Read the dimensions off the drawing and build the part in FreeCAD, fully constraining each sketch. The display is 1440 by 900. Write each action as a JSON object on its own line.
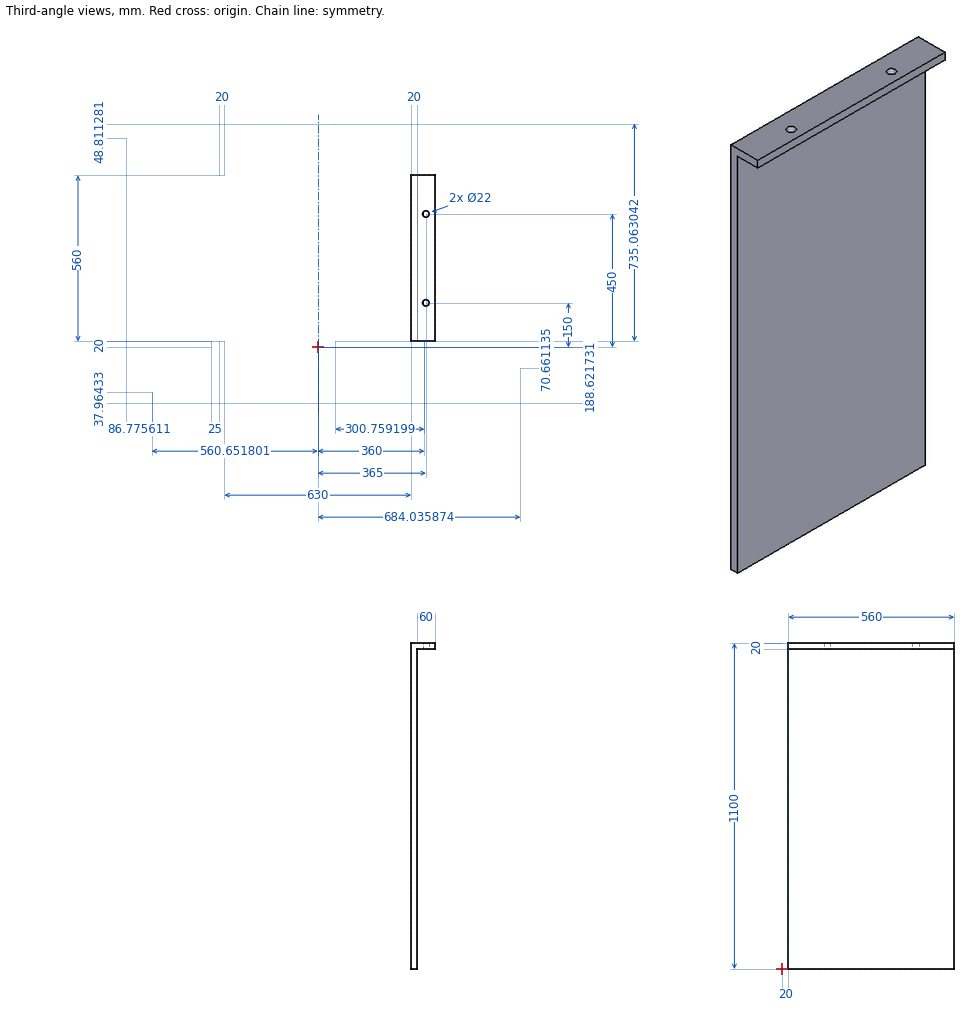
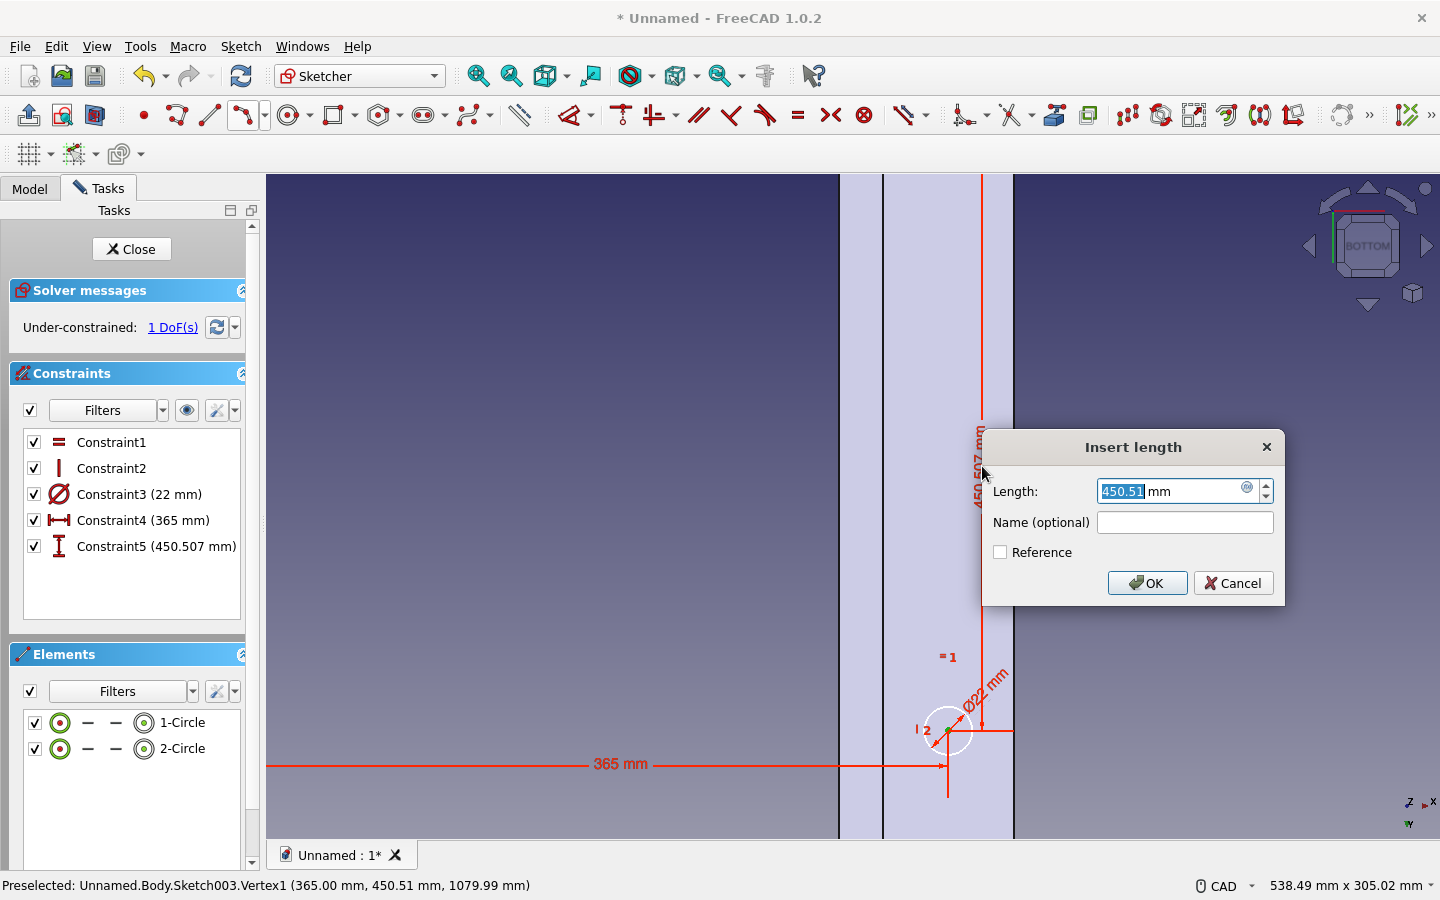
{"action": "type", "text": "450"}
{"action": "key", "text": "Return"}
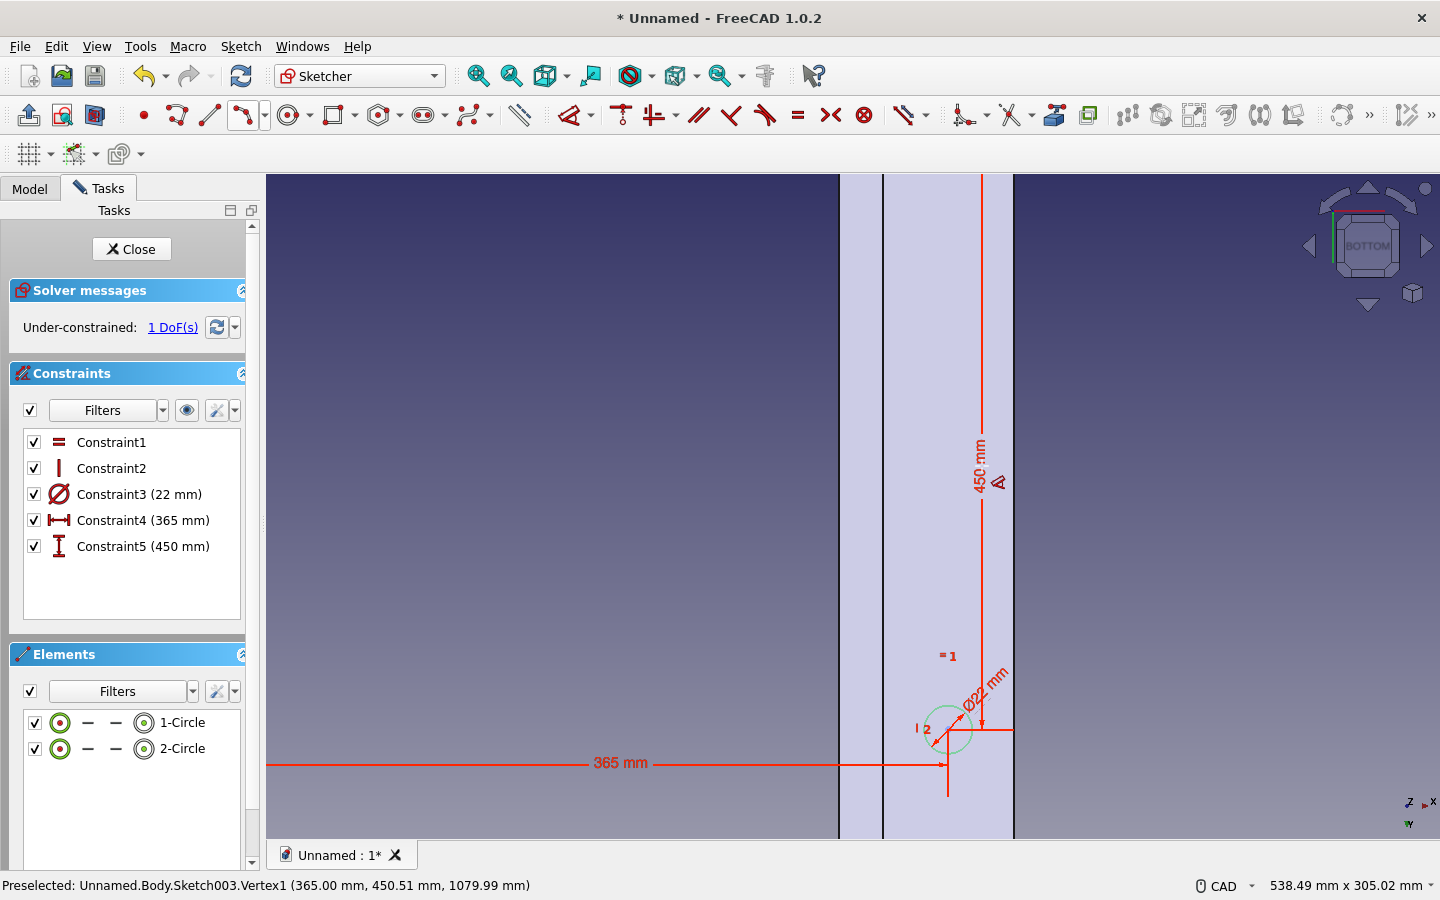
{"action": "scroll", "coordinate": [966, 715], "scroll_direction": "down", "scroll_amount": 4}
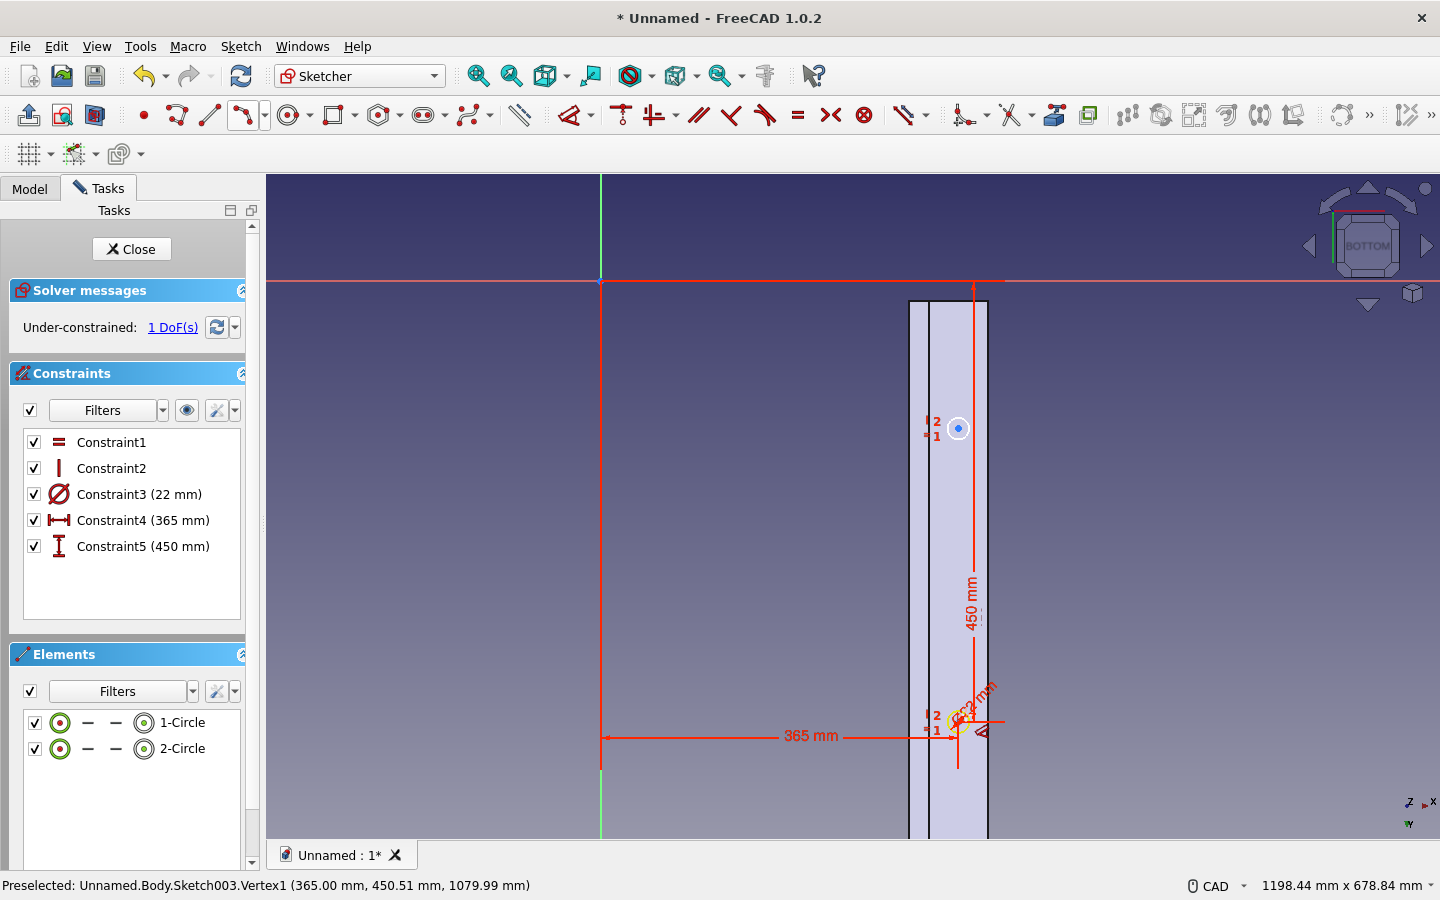
{"action": "left_click", "coordinate": [958, 429]}
{"action": "left_click", "coordinate": [567, 355]}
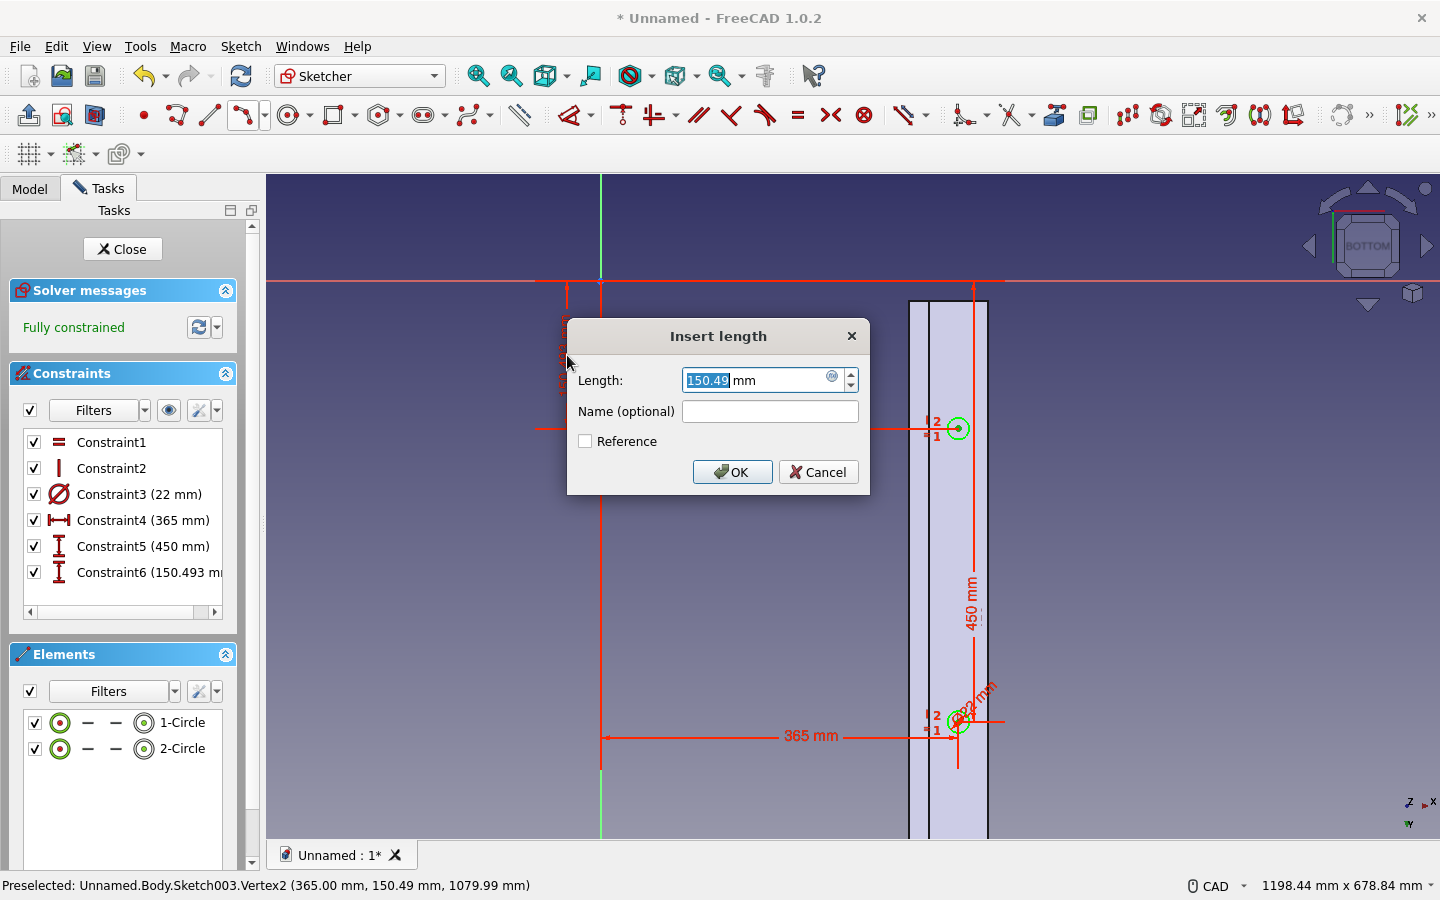
{"action": "type", "text": "150"}
{"action": "key", "text": "Return"}
{"action": "key", "text": "Escape"}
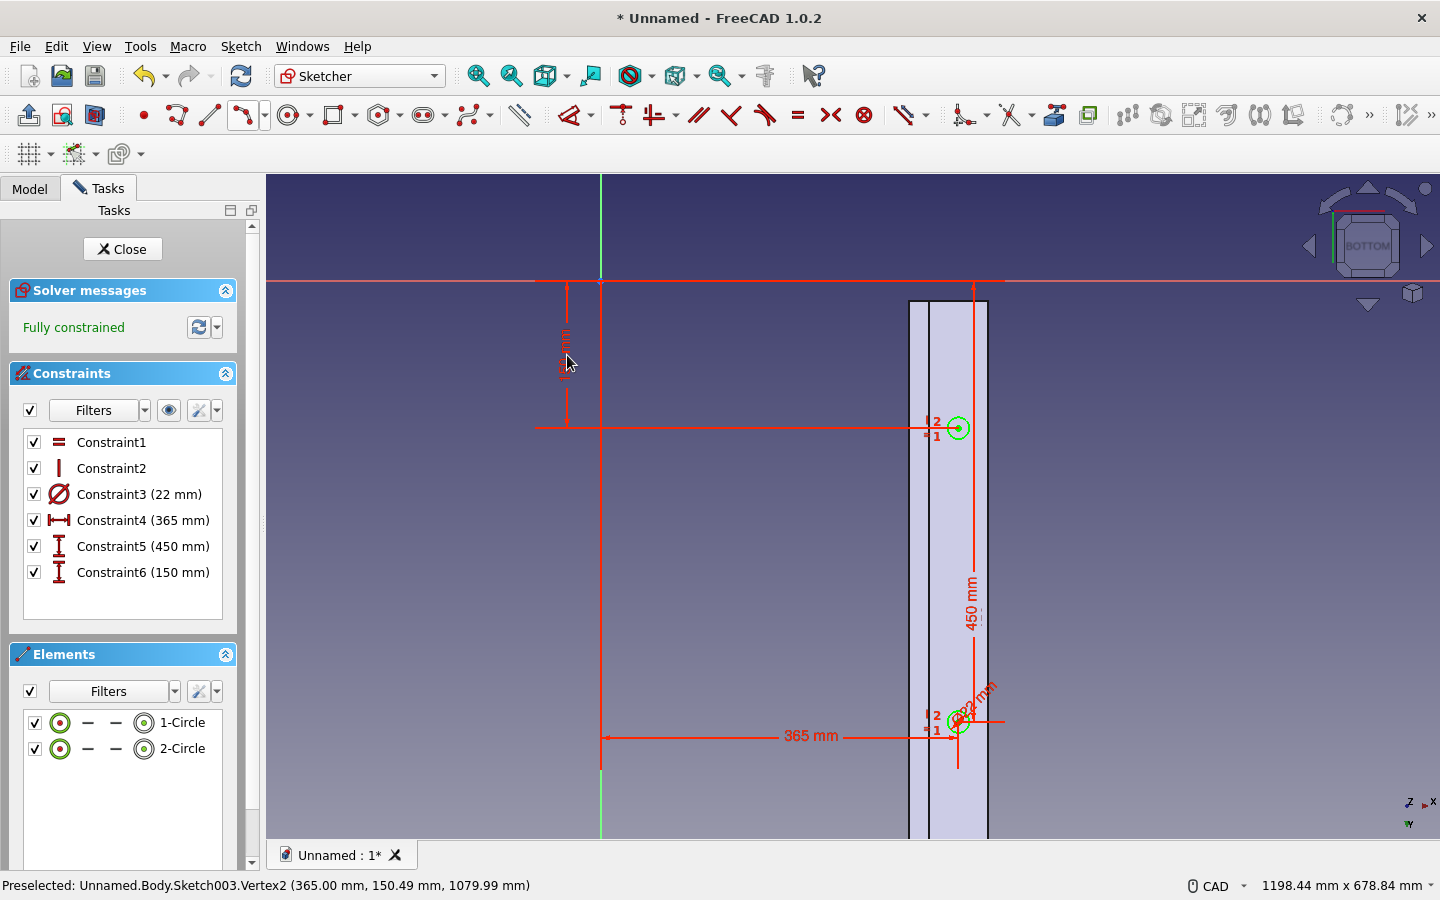
{"action": "left_click", "coordinate": [123, 249]}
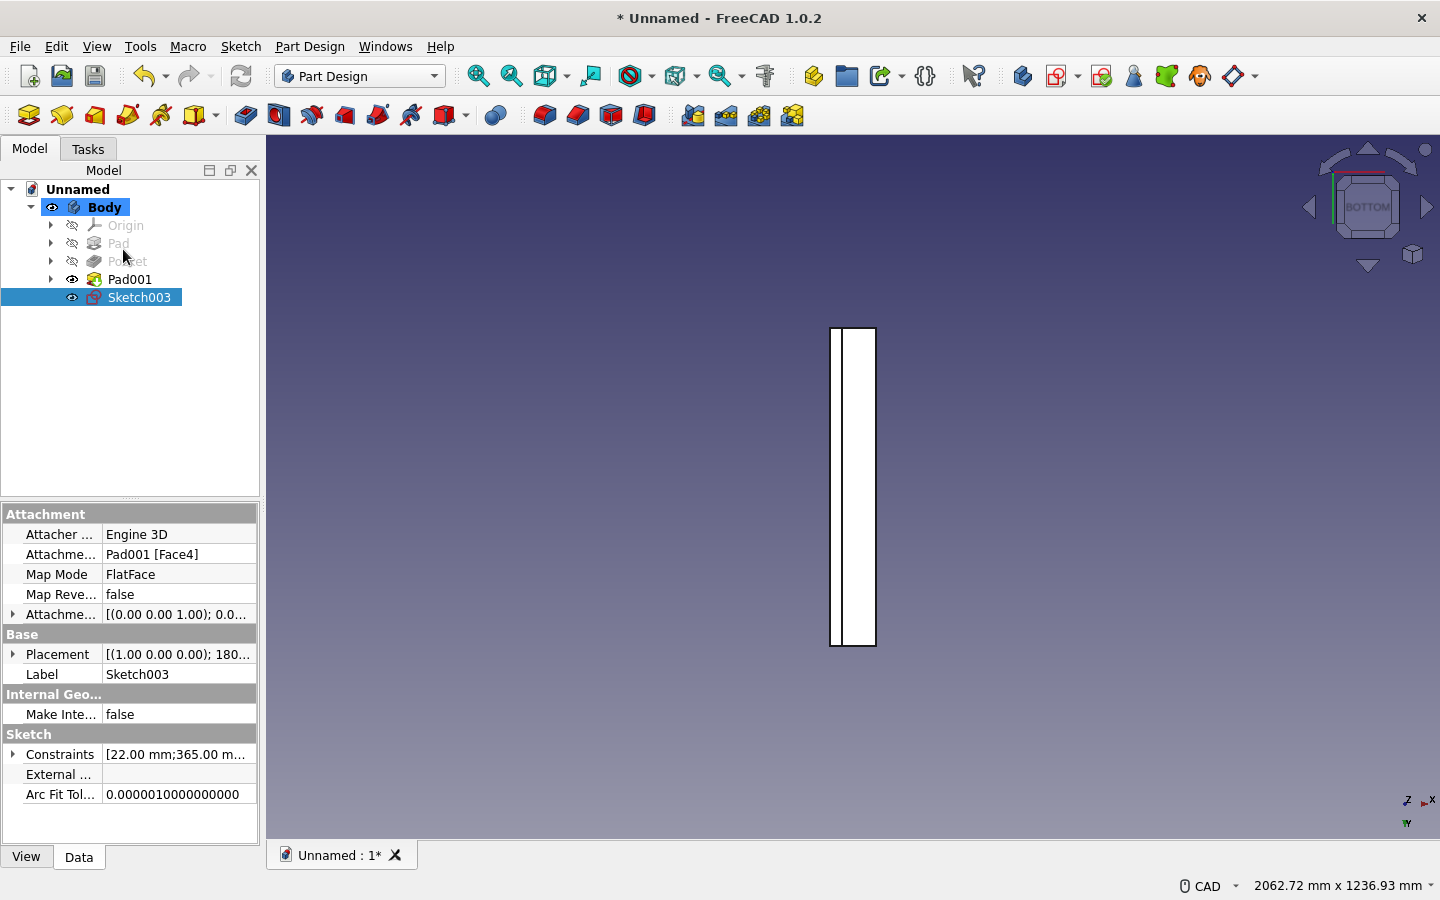
{"action": "left_click", "coordinate": [246, 116]}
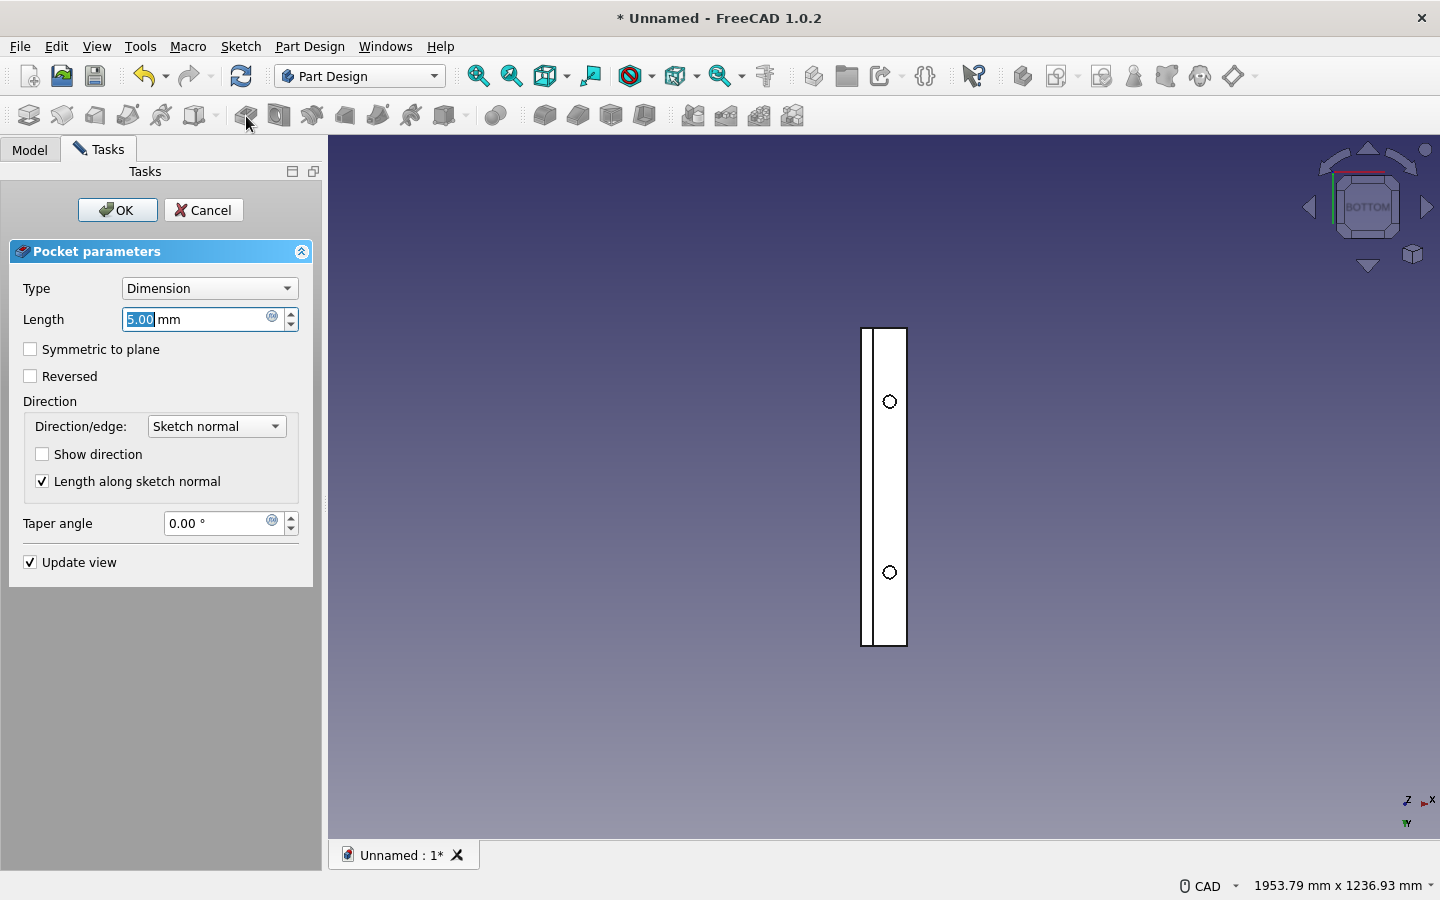
{"action": "left_click", "coordinate": [210, 288]}